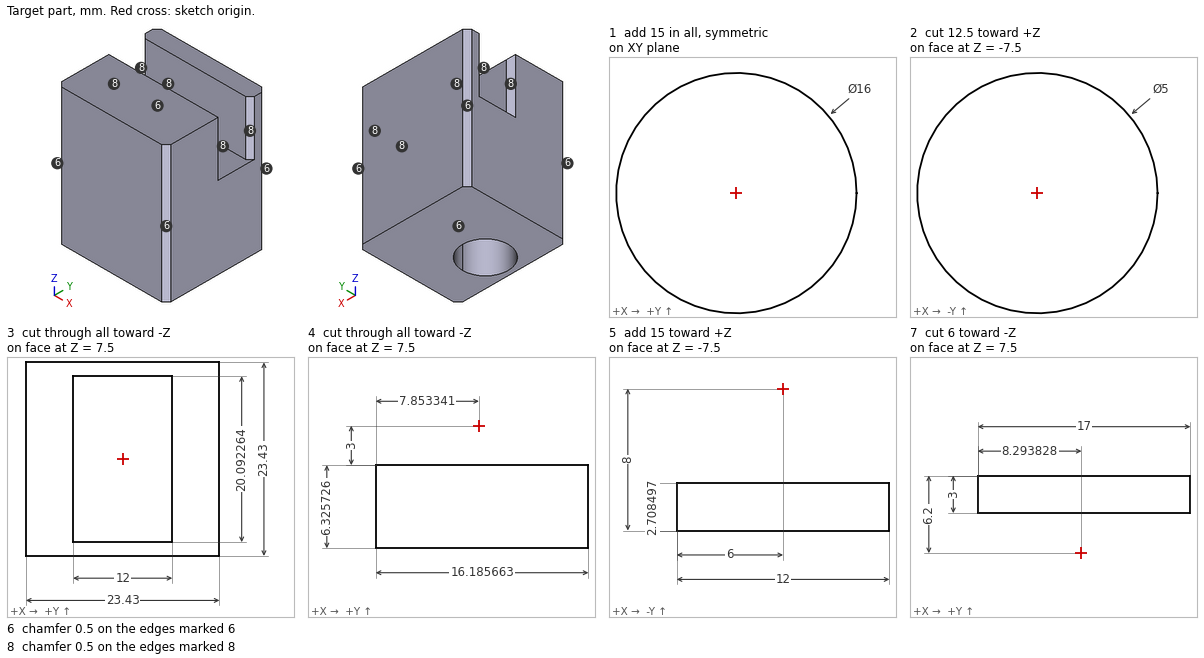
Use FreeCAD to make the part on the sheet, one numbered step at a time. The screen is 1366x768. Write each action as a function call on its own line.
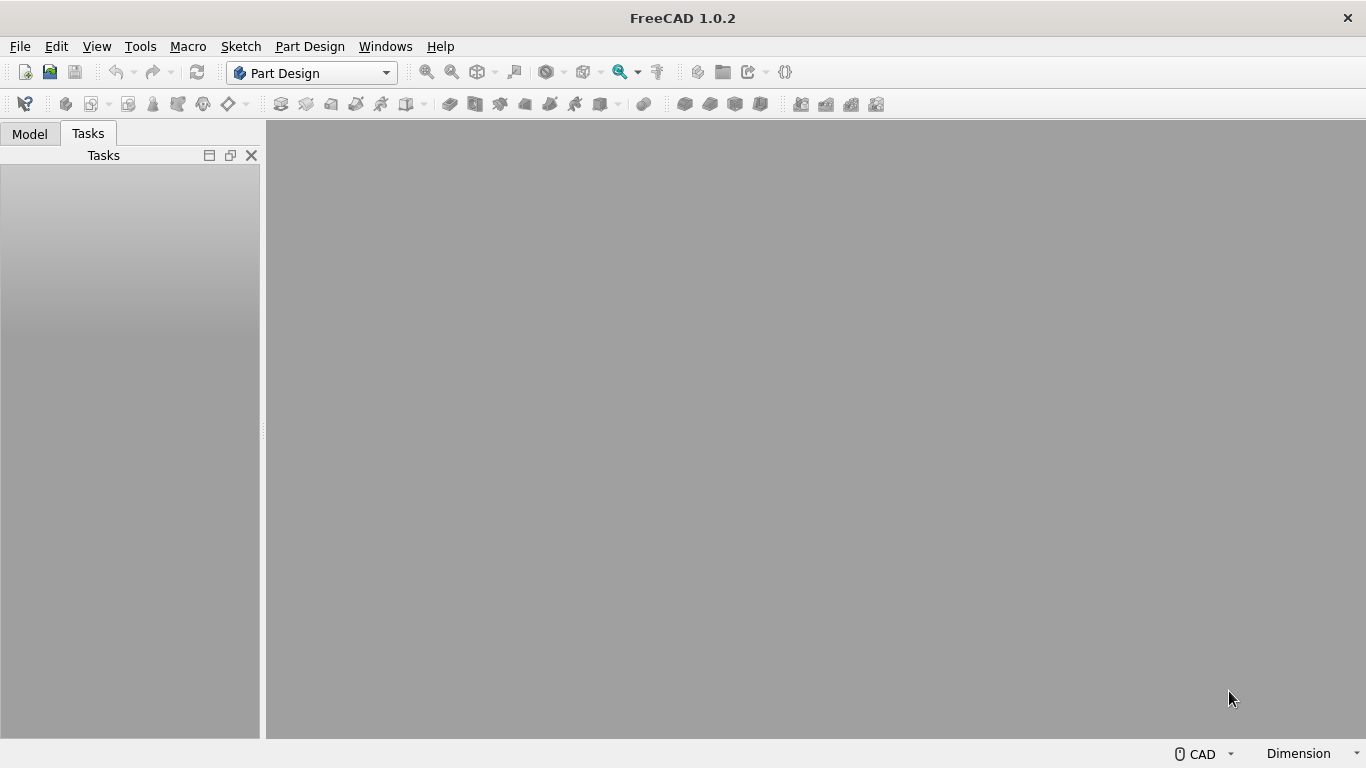
click(25, 72)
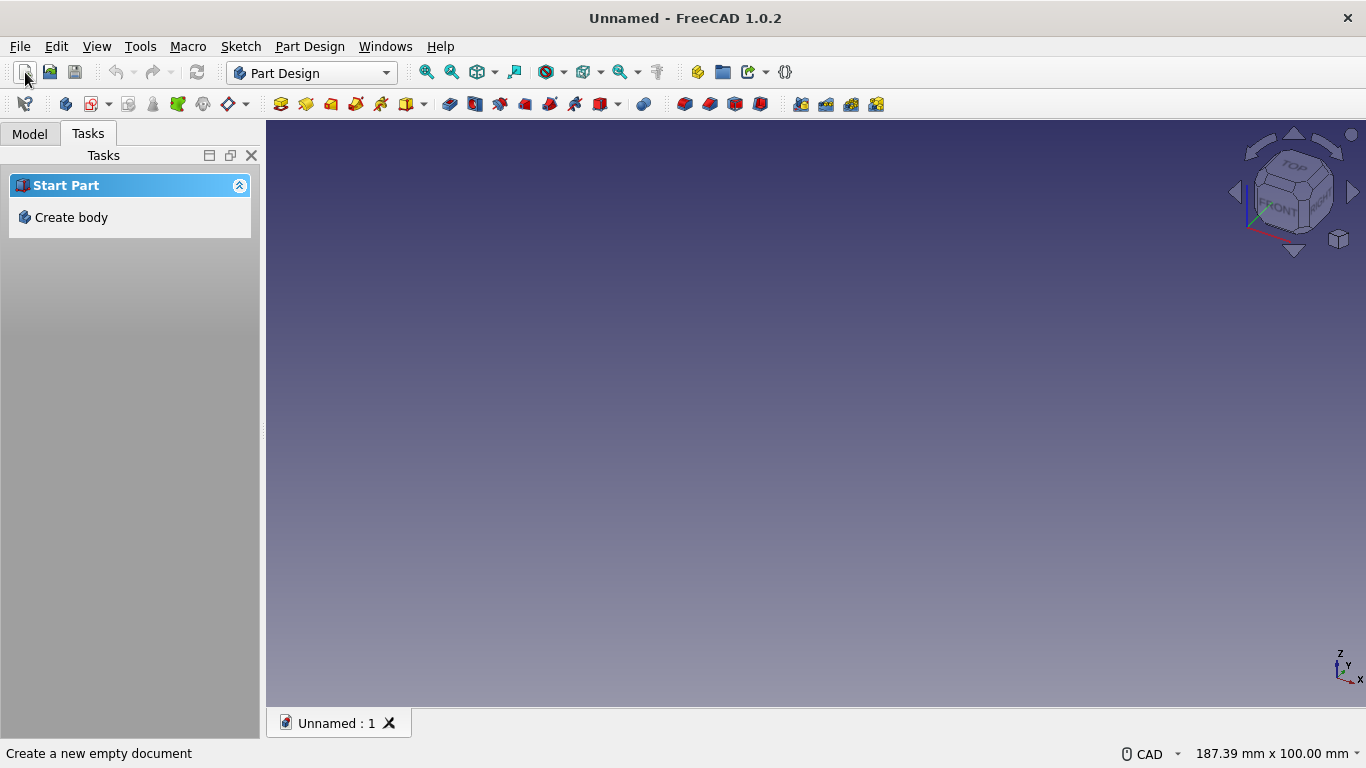
click(90, 104)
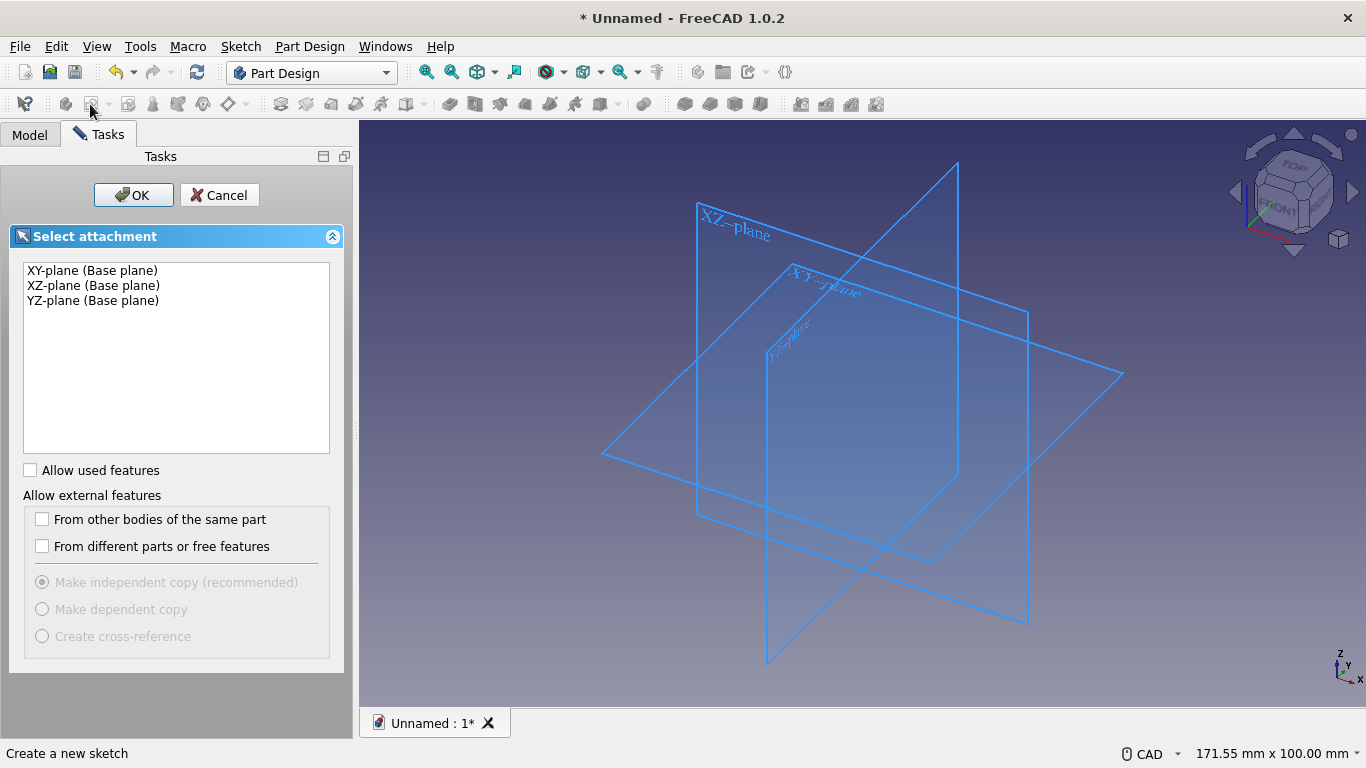
click(84, 270)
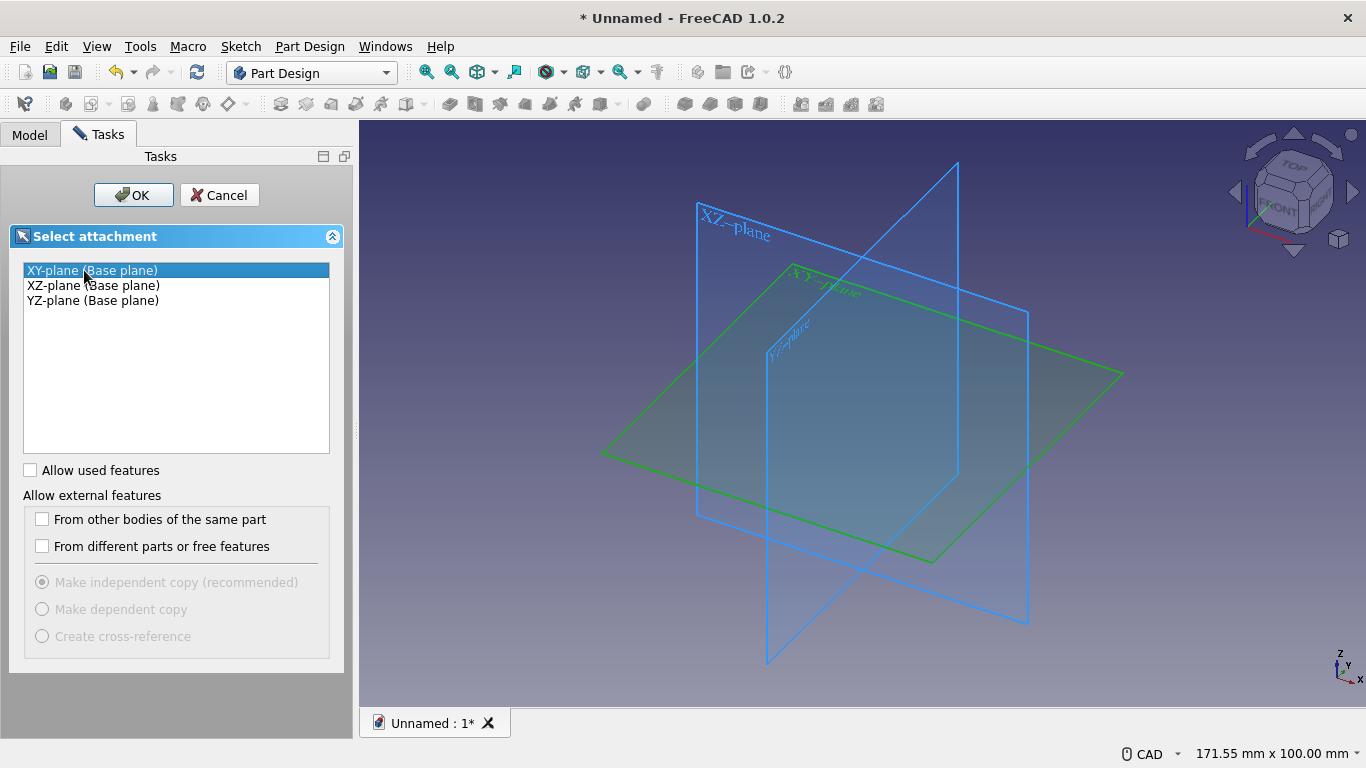
click(134, 195)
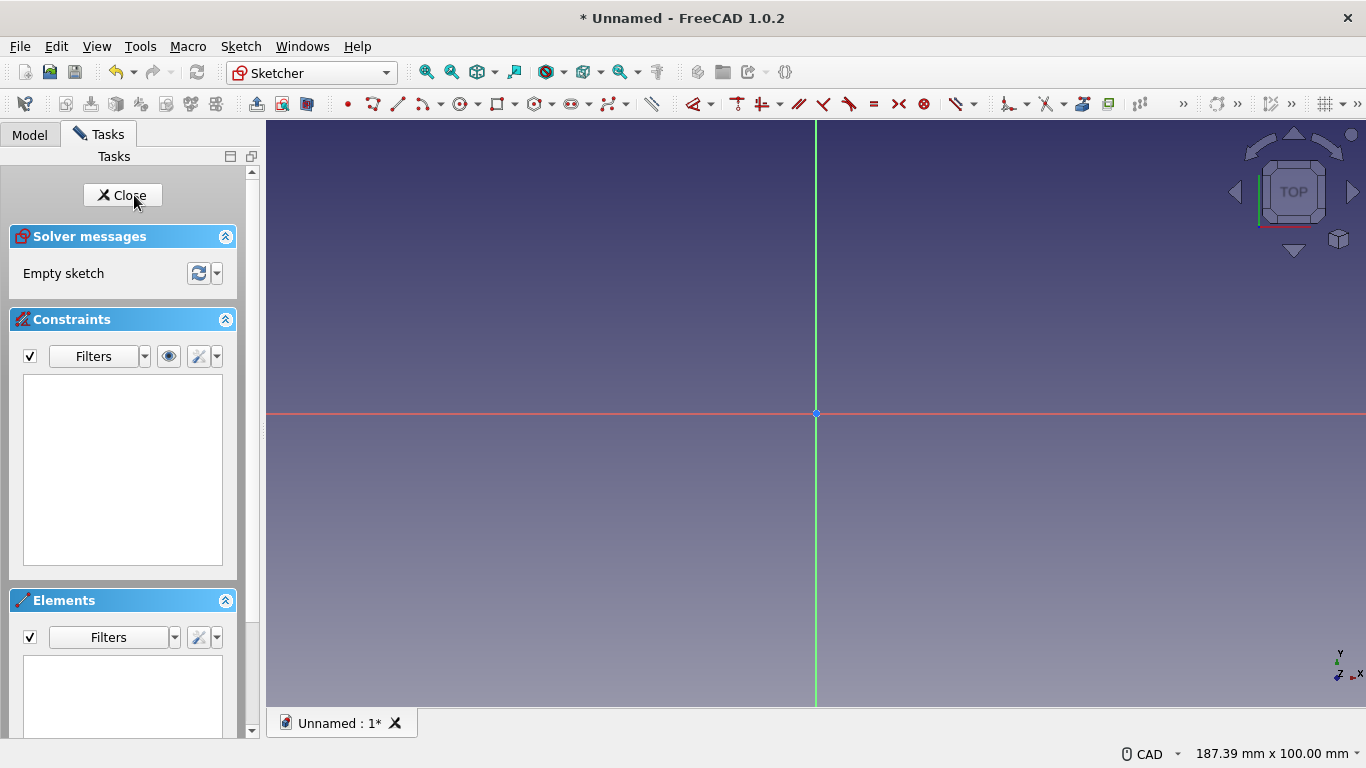
scroll(838, 414, up, 7)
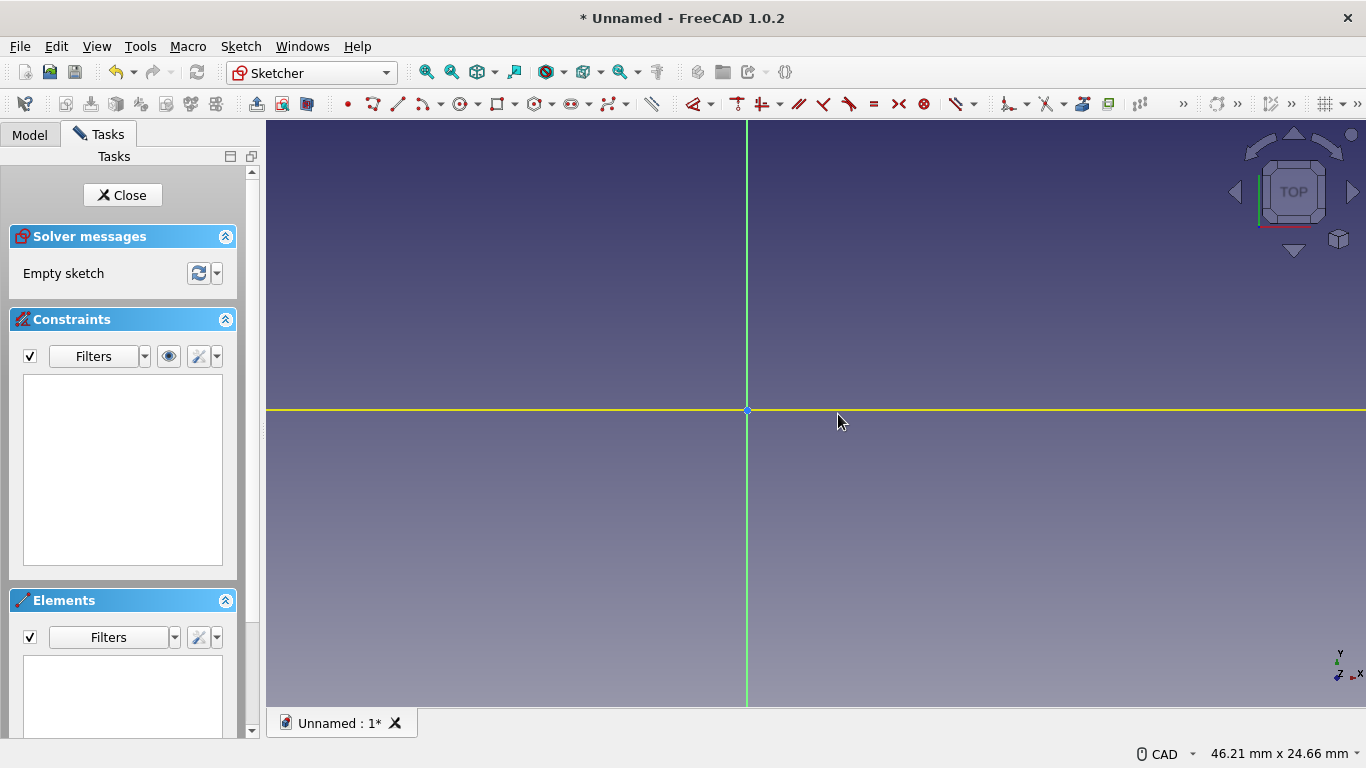
click(460, 104)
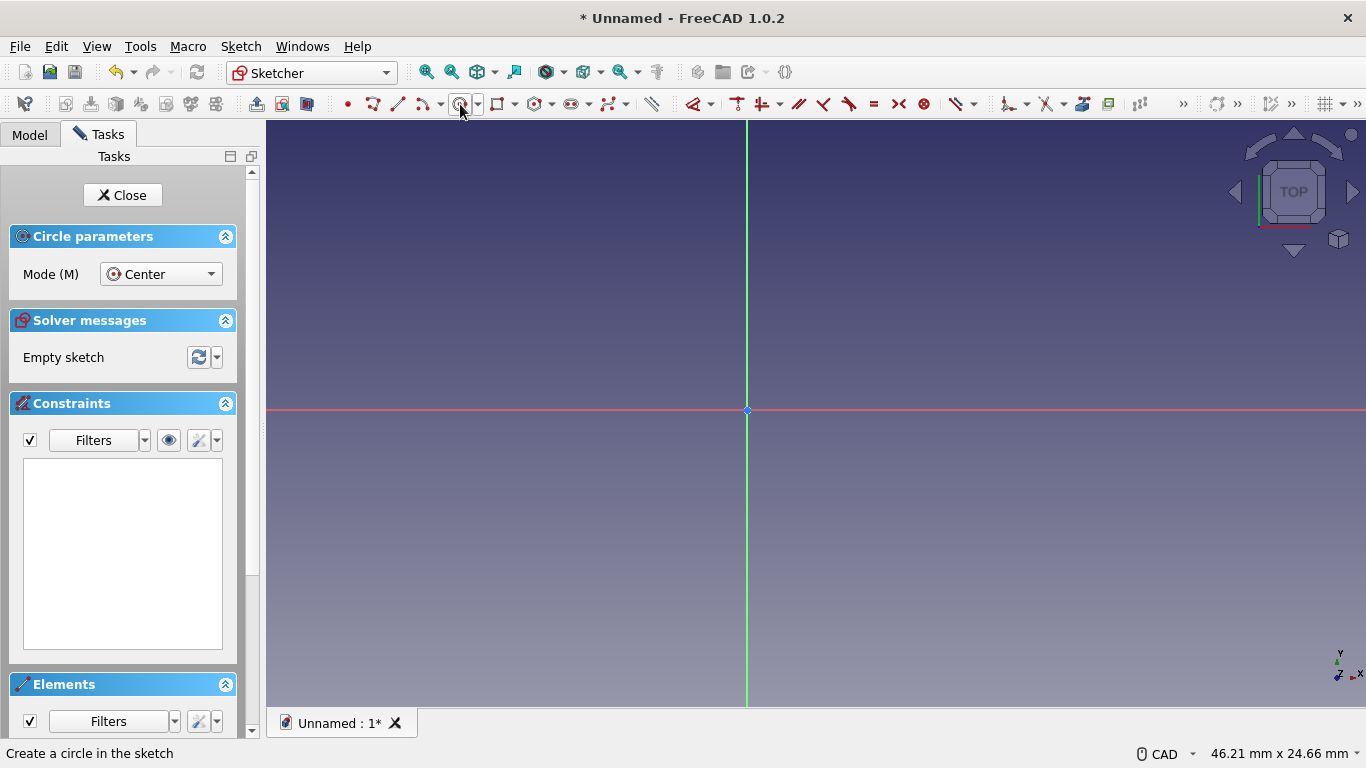
click(747, 410)
click(882, 276)
key(Escape)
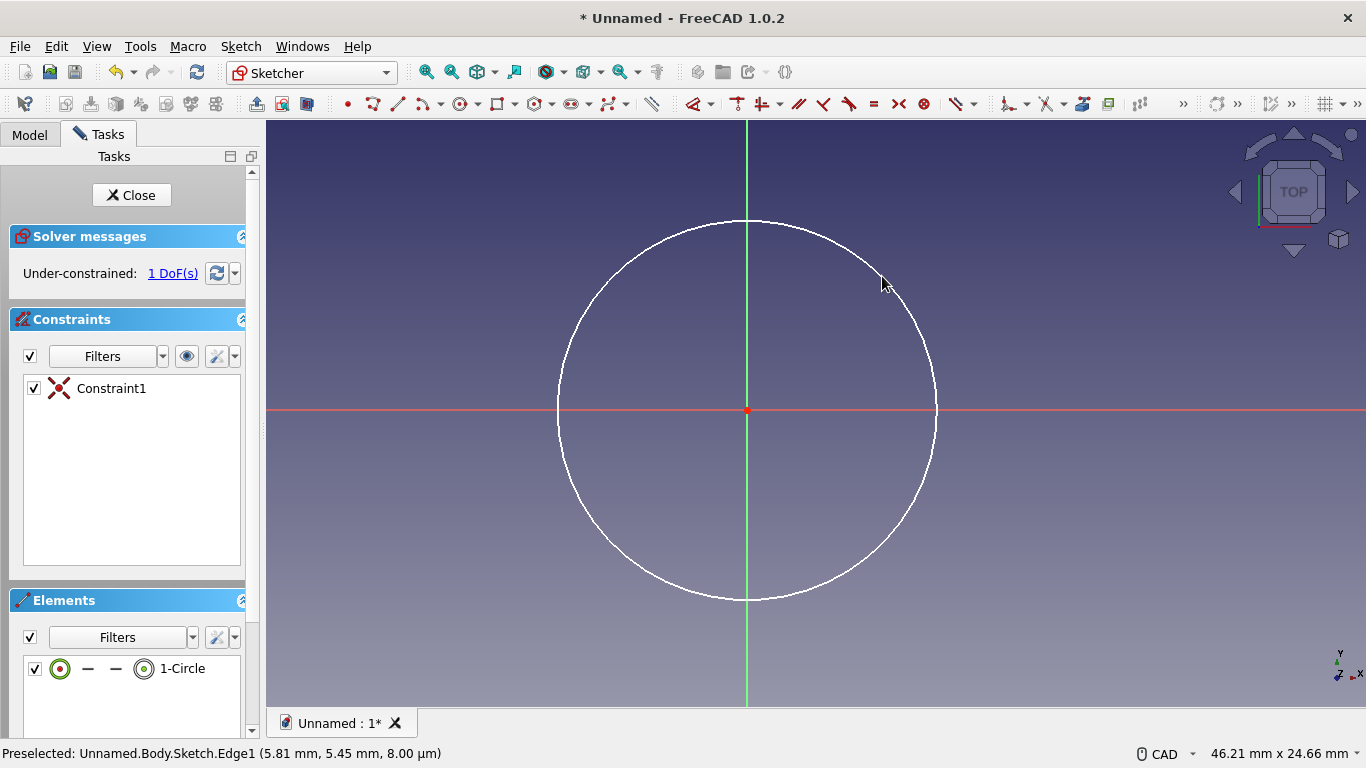
click(692, 104)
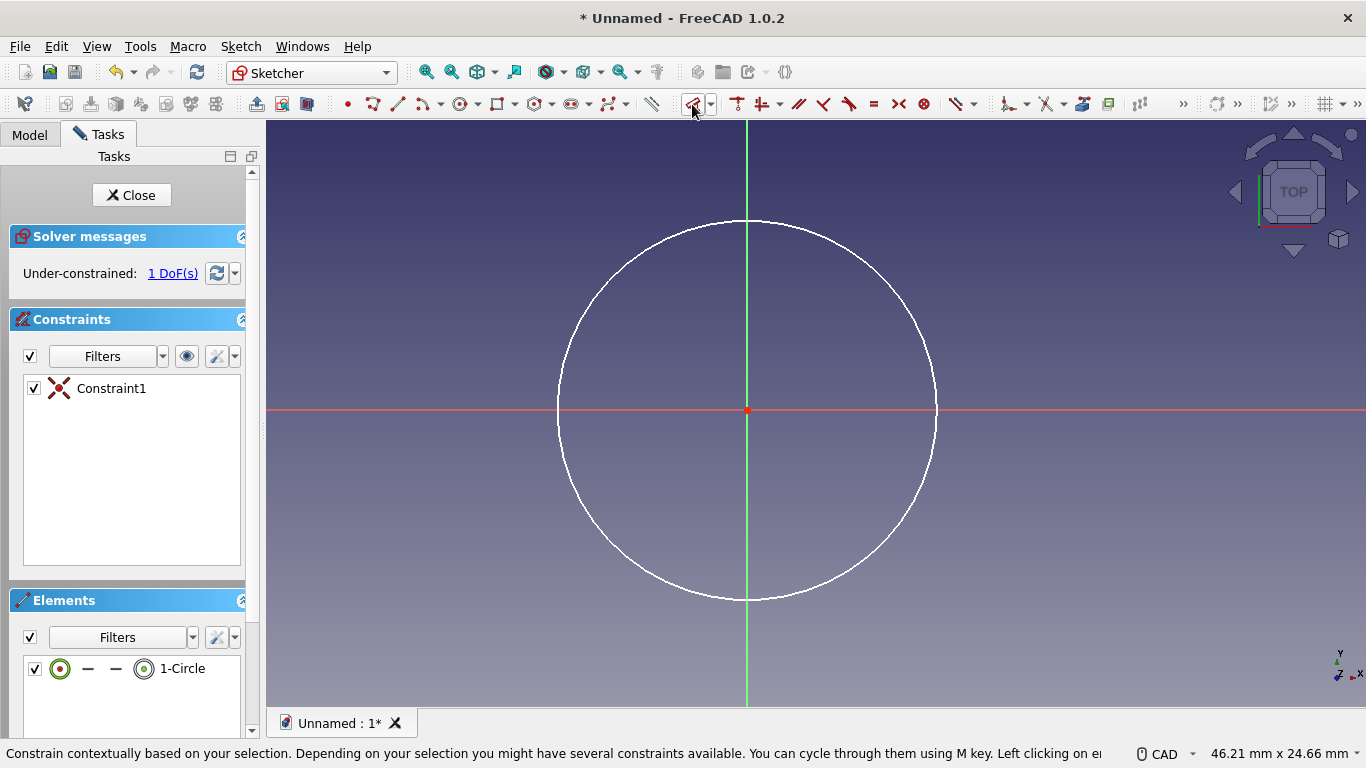
click(881, 276)
click(904, 253)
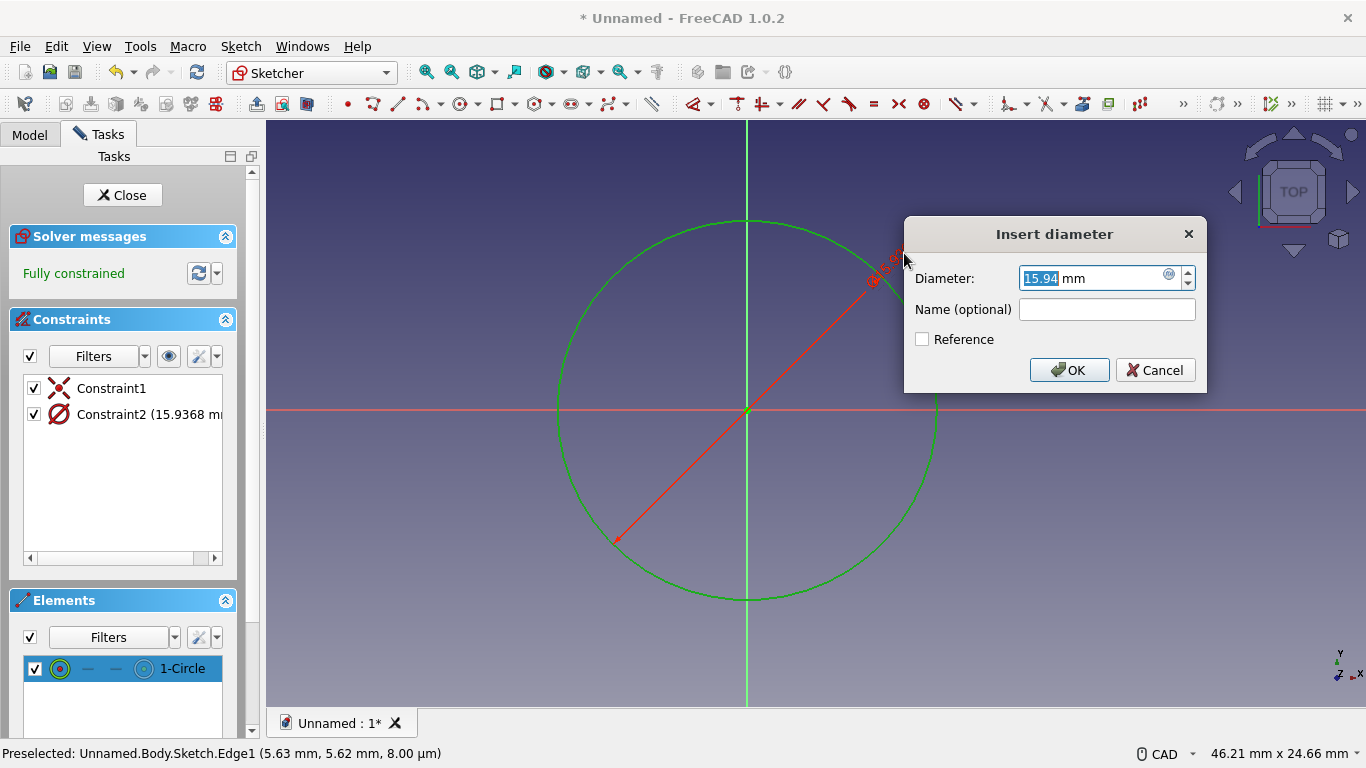
text(16)
key(Return)
key(Escape)